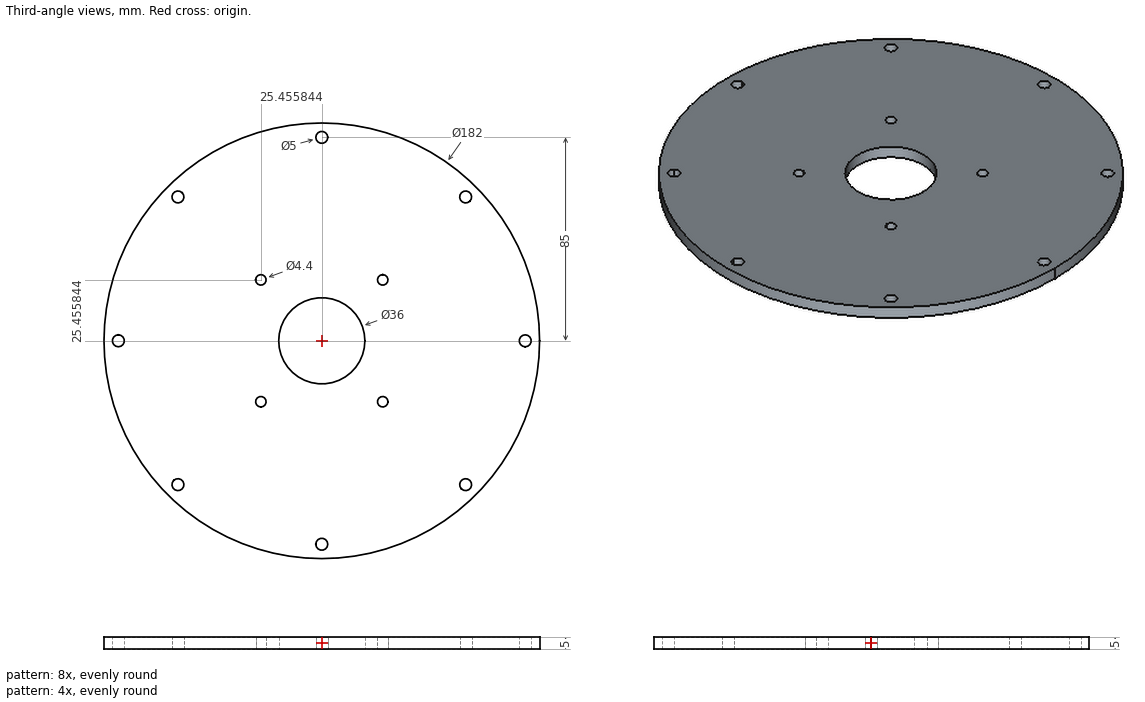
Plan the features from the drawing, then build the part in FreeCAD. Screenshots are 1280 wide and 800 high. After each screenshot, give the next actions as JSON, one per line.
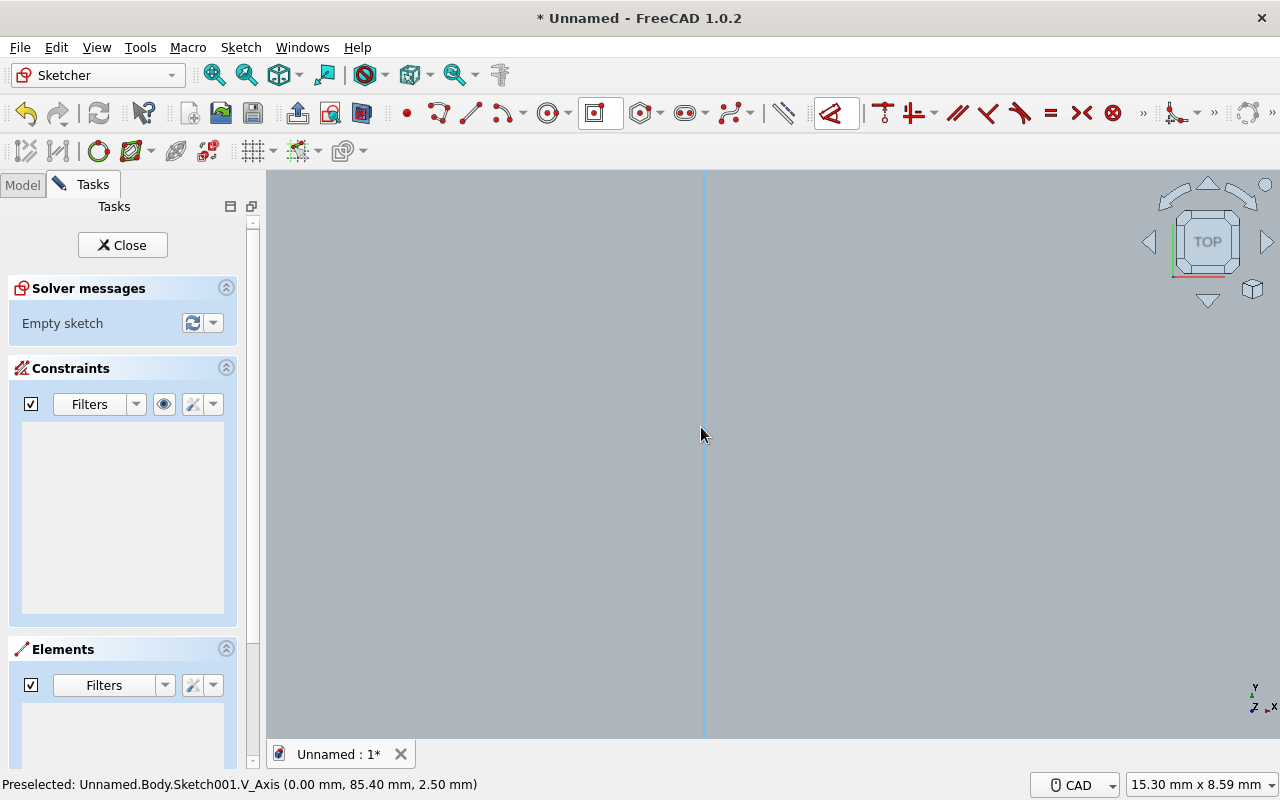
{"action": "left_click", "coordinate": [548, 114]}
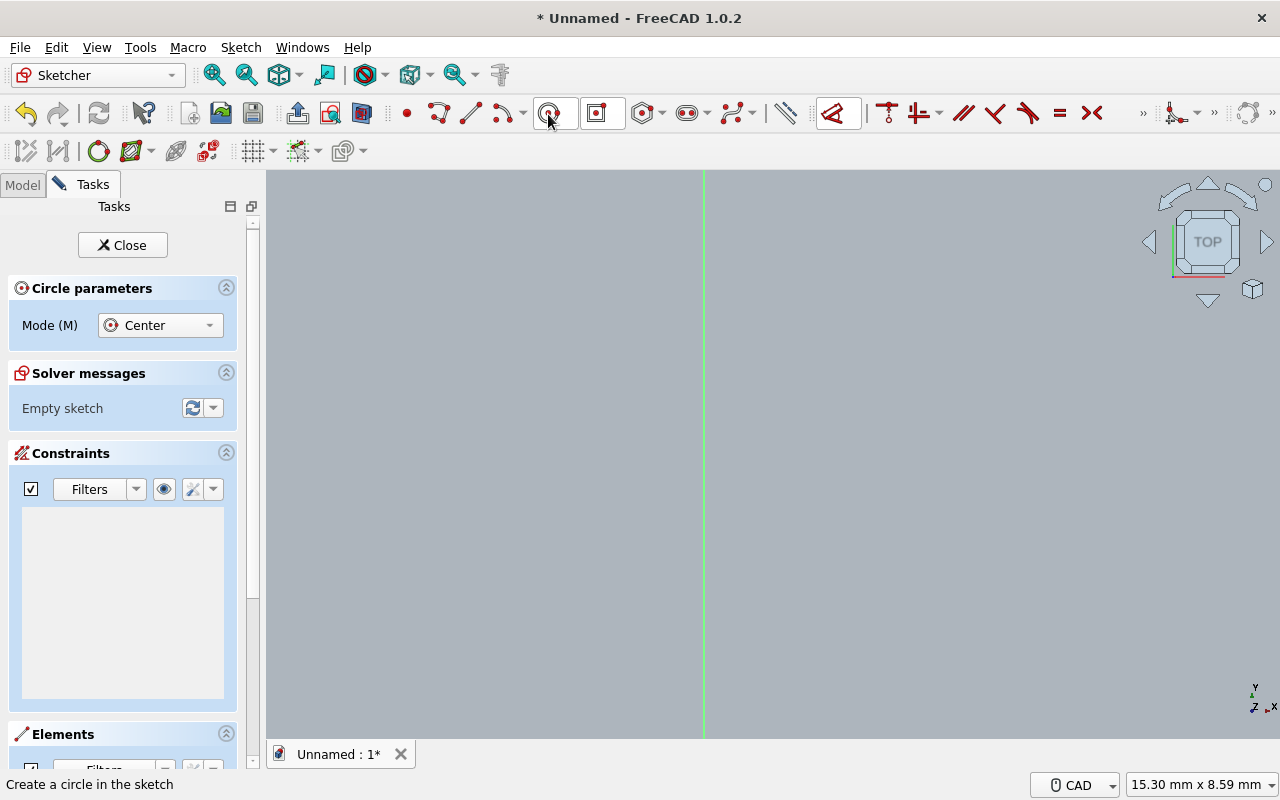
{"action": "left_click", "coordinate": [704, 454]}
{"action": "mouse_move", "coordinate": [822, 337]}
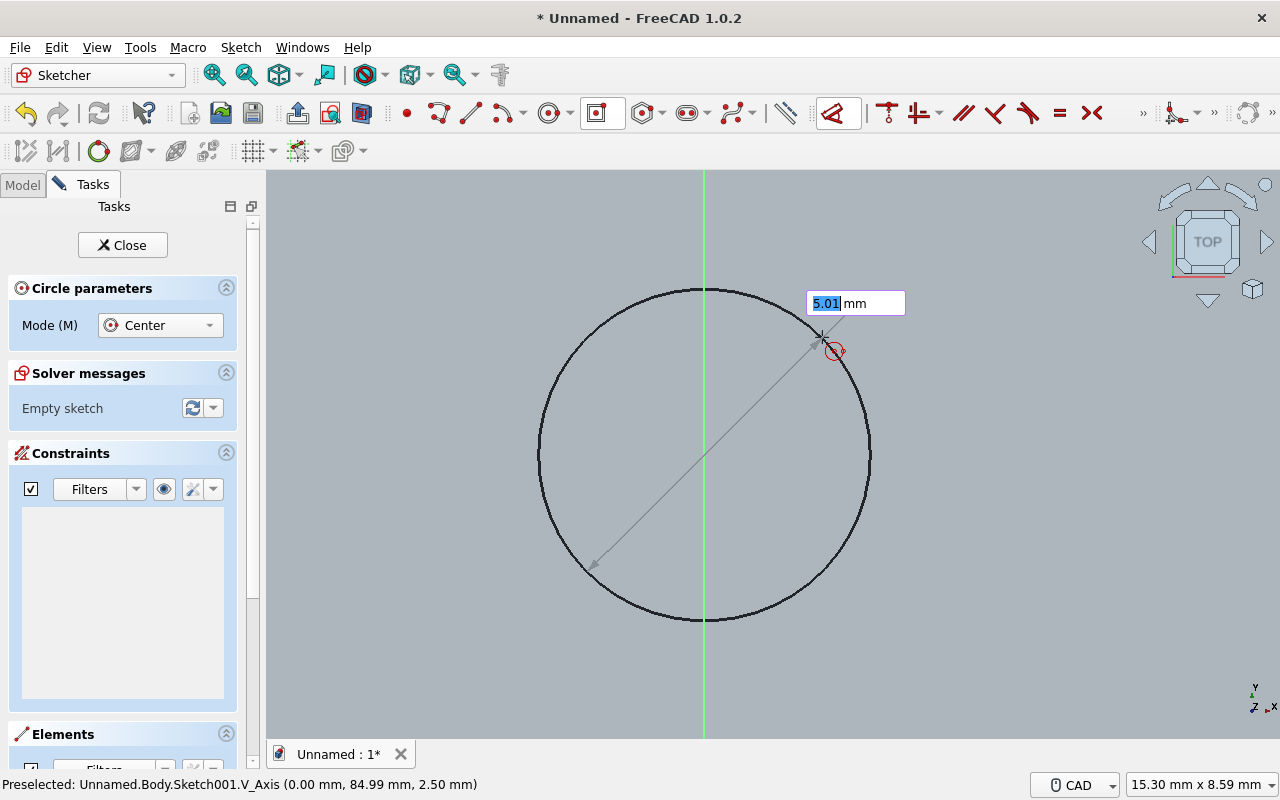
{"action": "type", "text": "5"}
{"action": "key", "text": "Return"}
{"action": "key", "text": "Escape"}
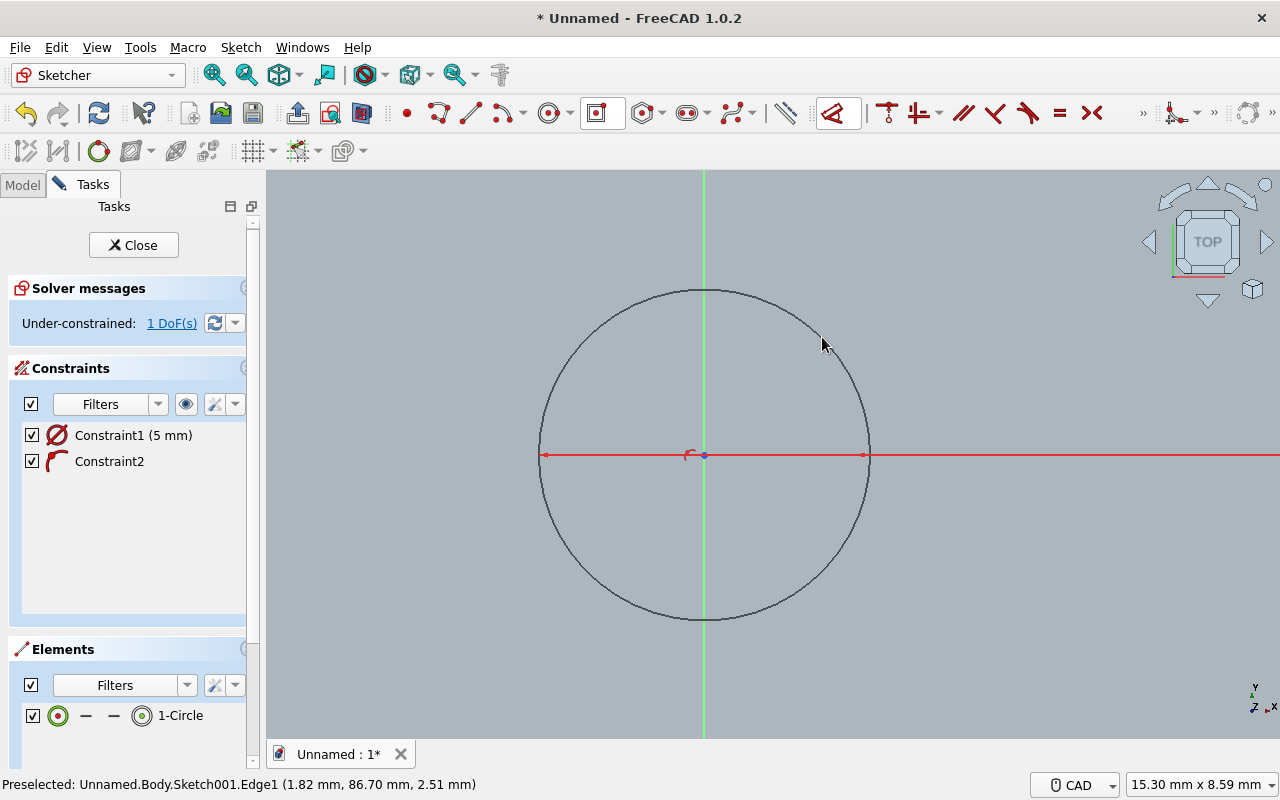
{"action": "left_click", "coordinate": [832, 114]}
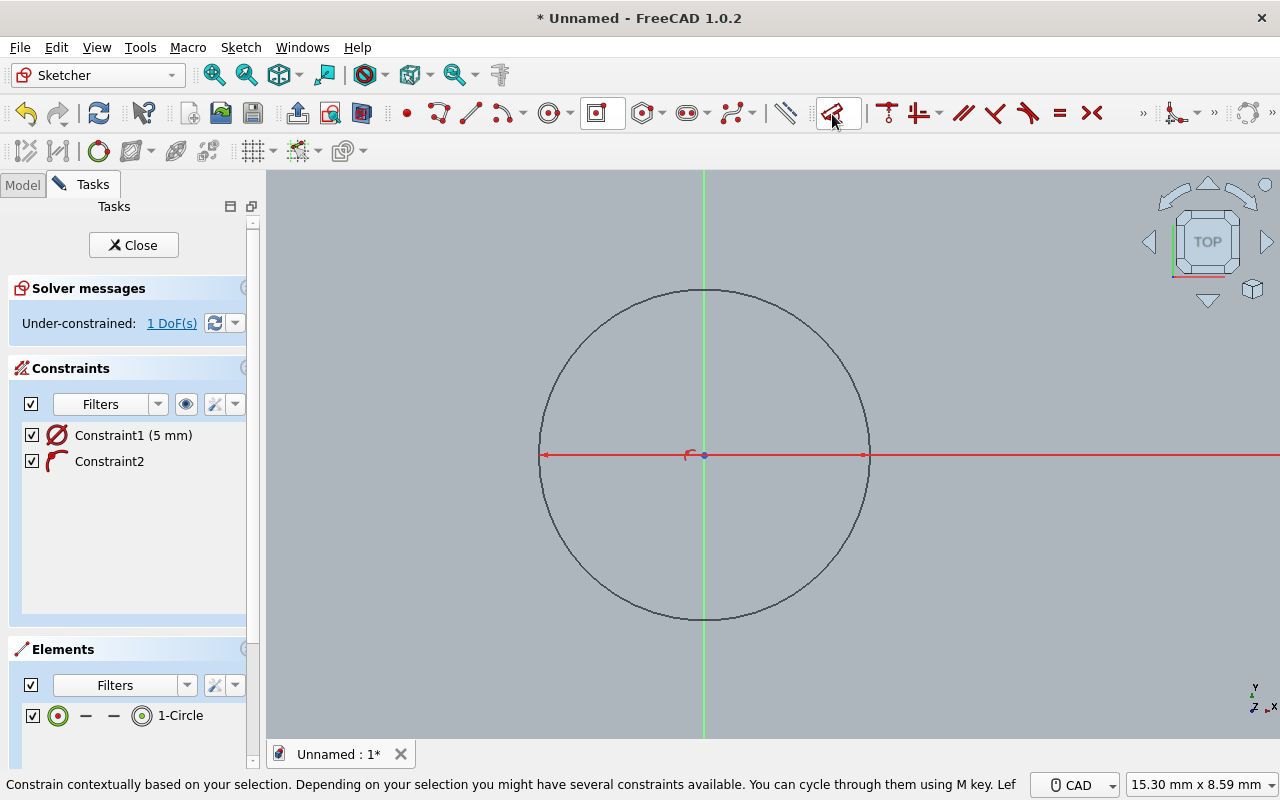
{"action": "left_click", "coordinate": [704, 455]}
{"action": "left_click", "coordinate": [738, 583]}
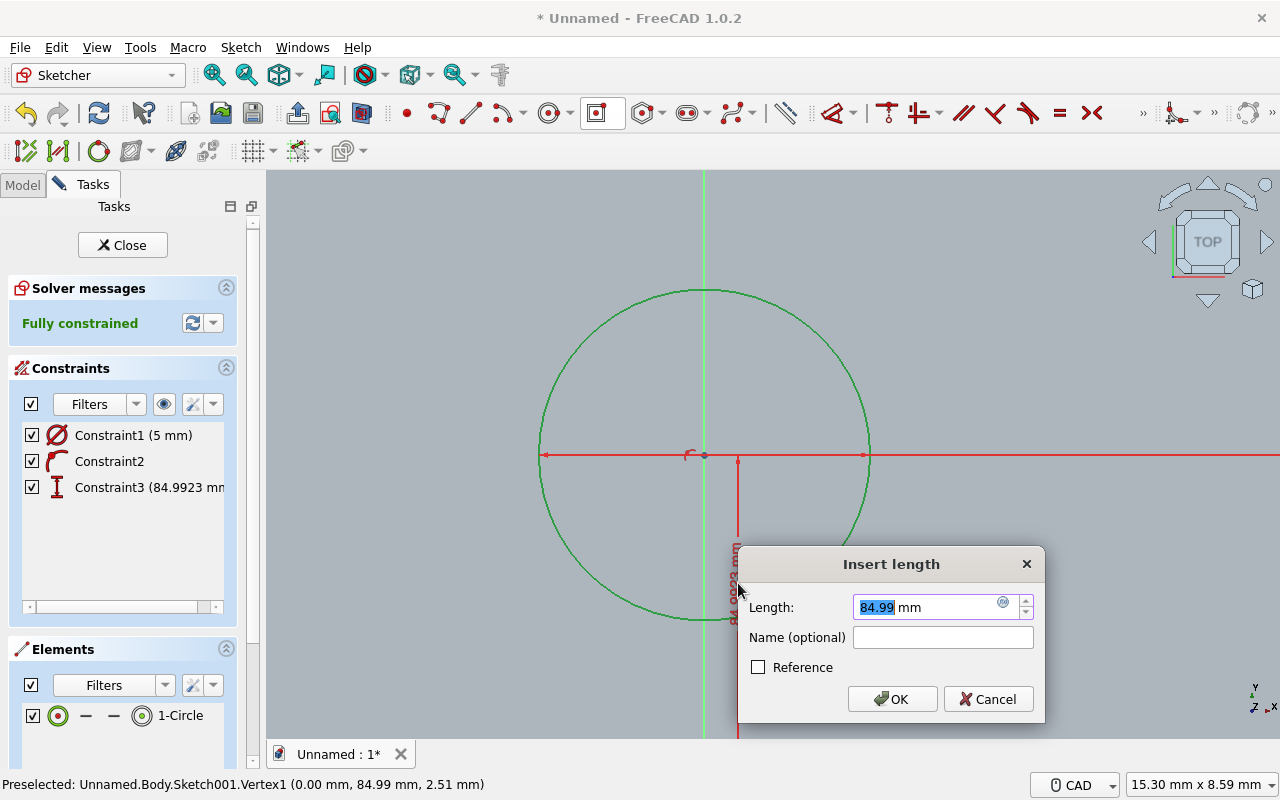
{"action": "type", "text": "85"}
{"action": "key", "text": "Return"}
{"action": "key", "text": "Escape"}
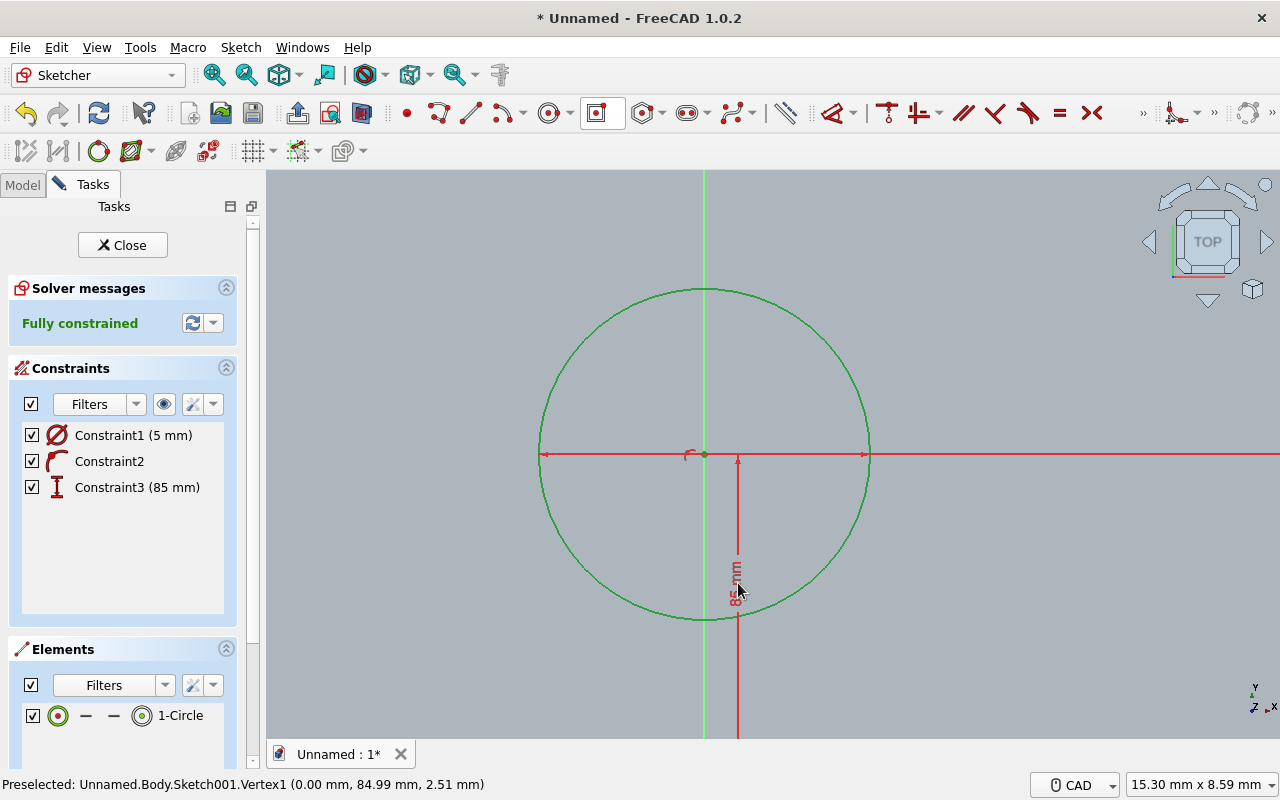
{"action": "left_click", "coordinate": [123, 245]}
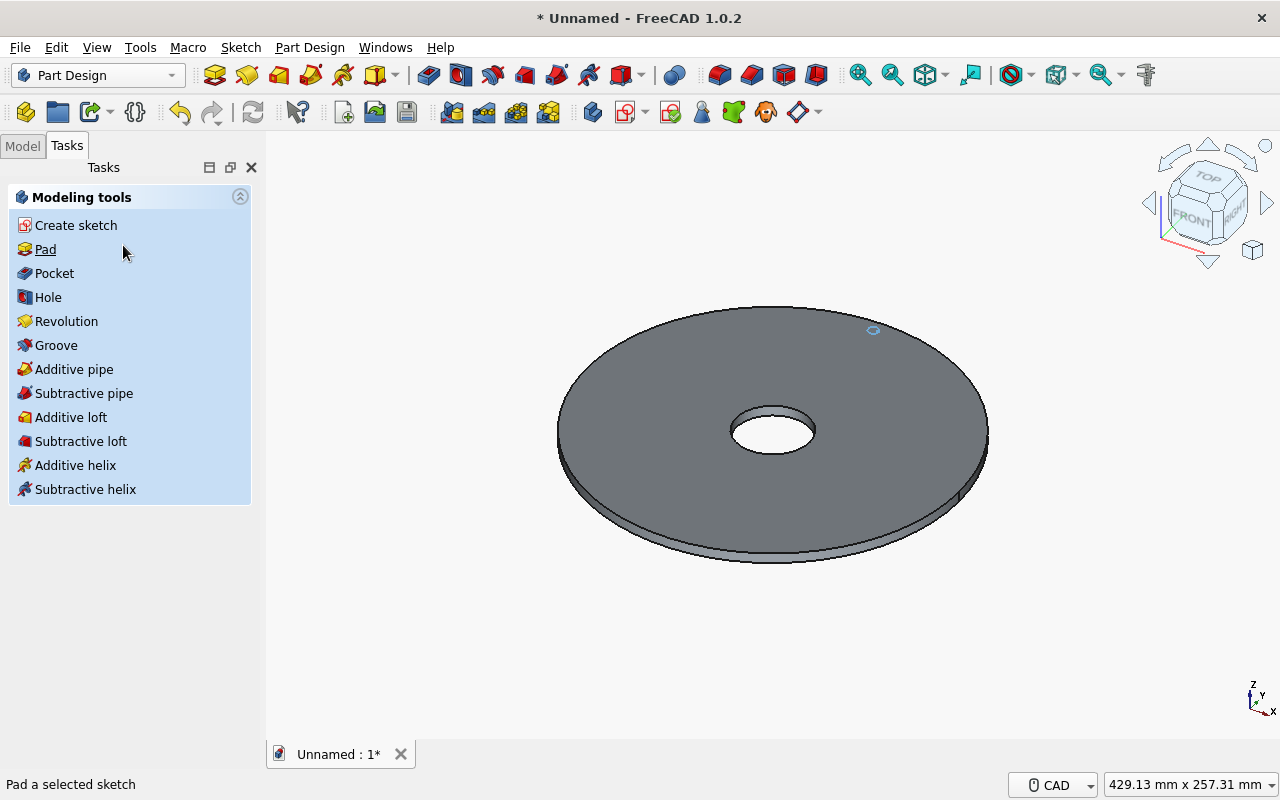
{"action": "left_click", "coordinate": [430, 76]}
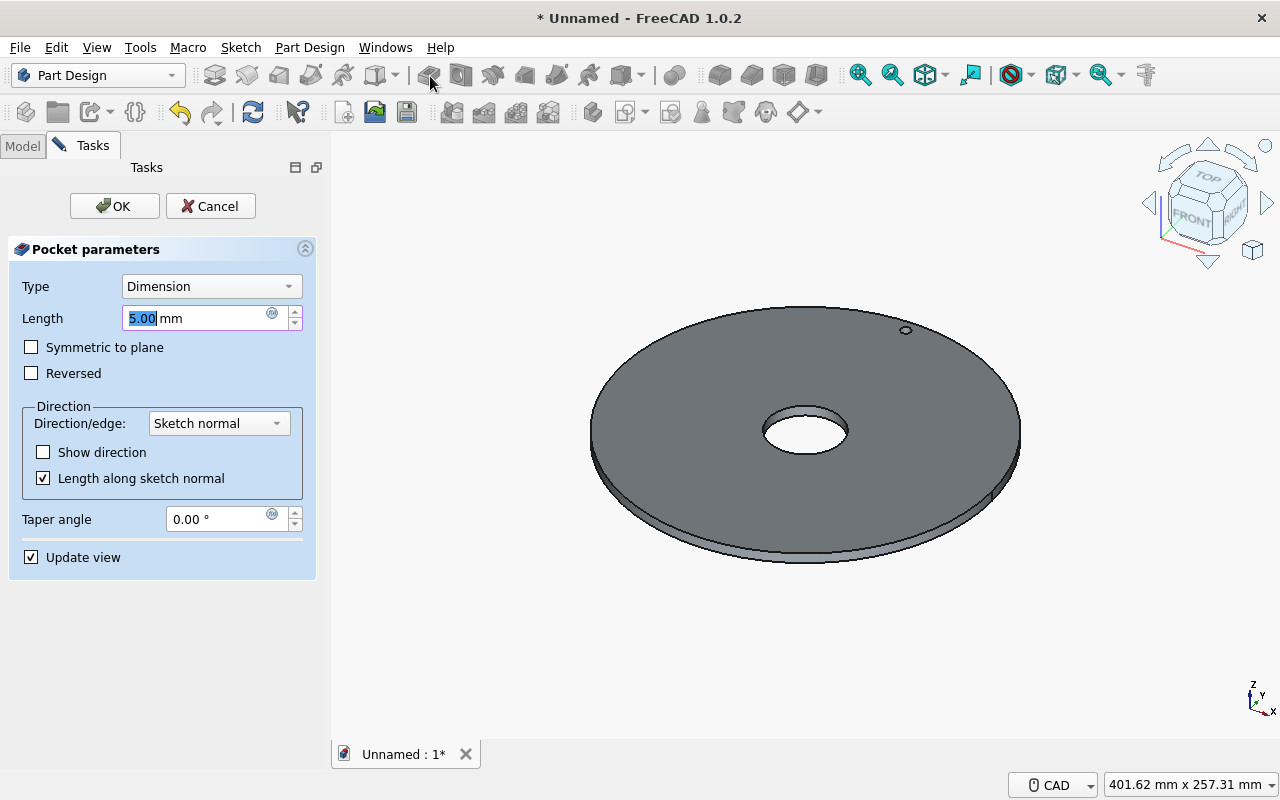
{"action": "type", "text": "5"}
{"action": "key", "text": "Tab"}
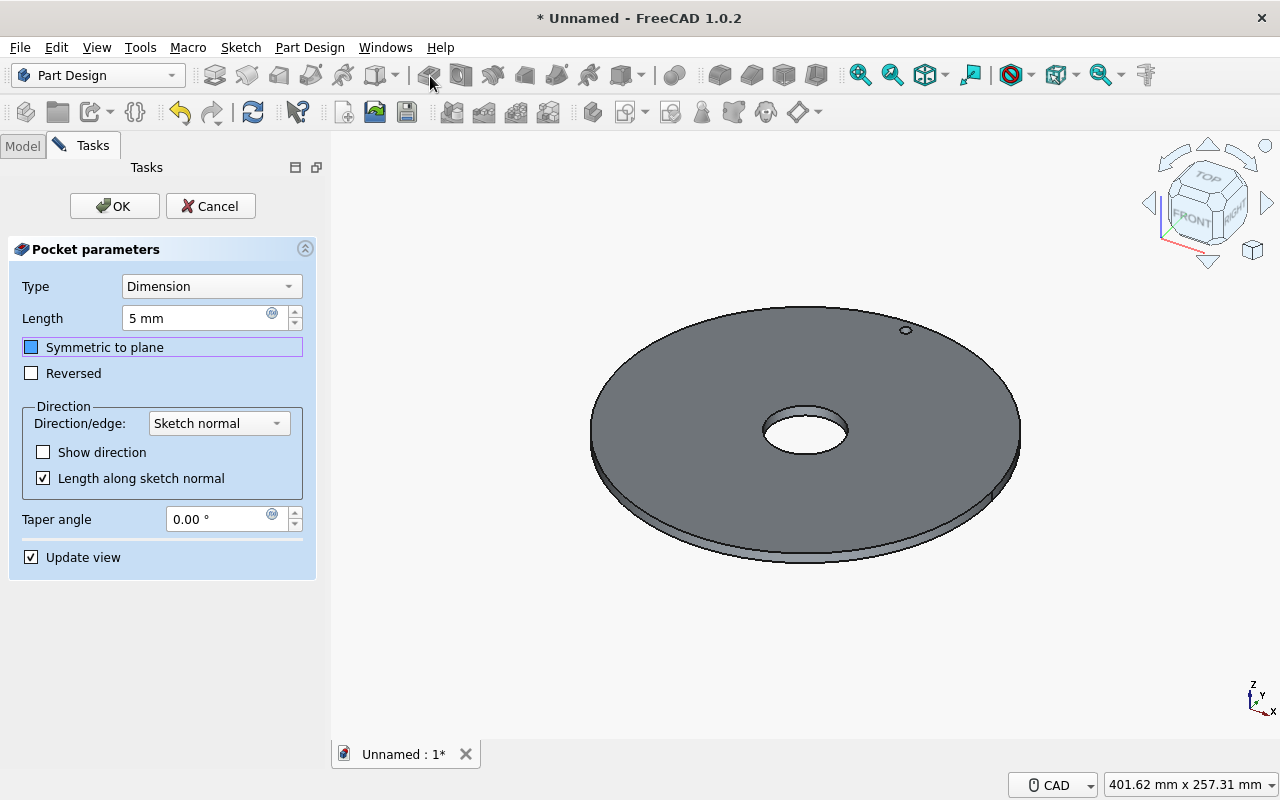
{"action": "left_click", "coordinate": [115, 206]}